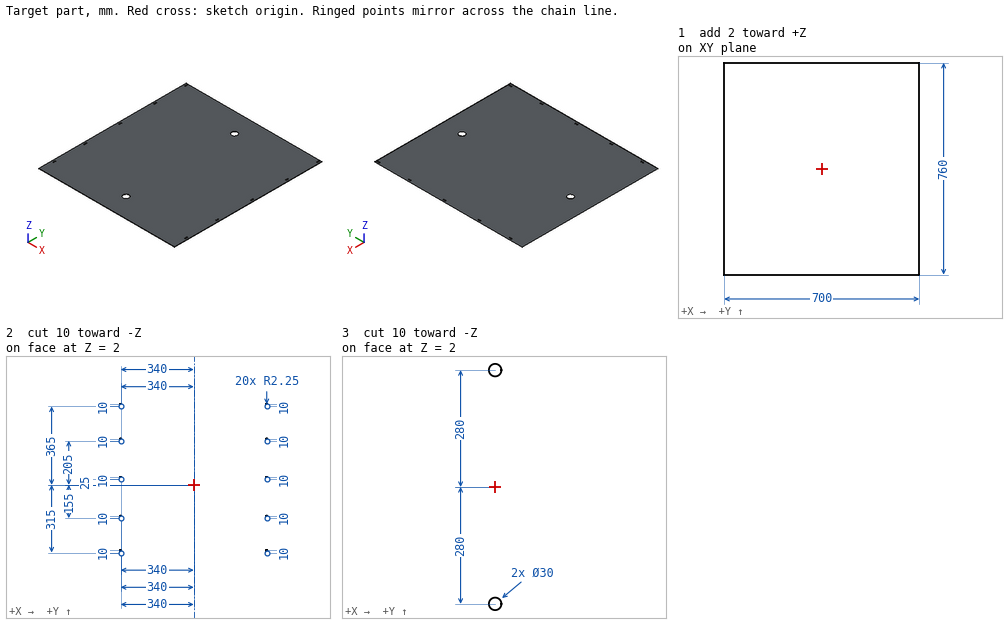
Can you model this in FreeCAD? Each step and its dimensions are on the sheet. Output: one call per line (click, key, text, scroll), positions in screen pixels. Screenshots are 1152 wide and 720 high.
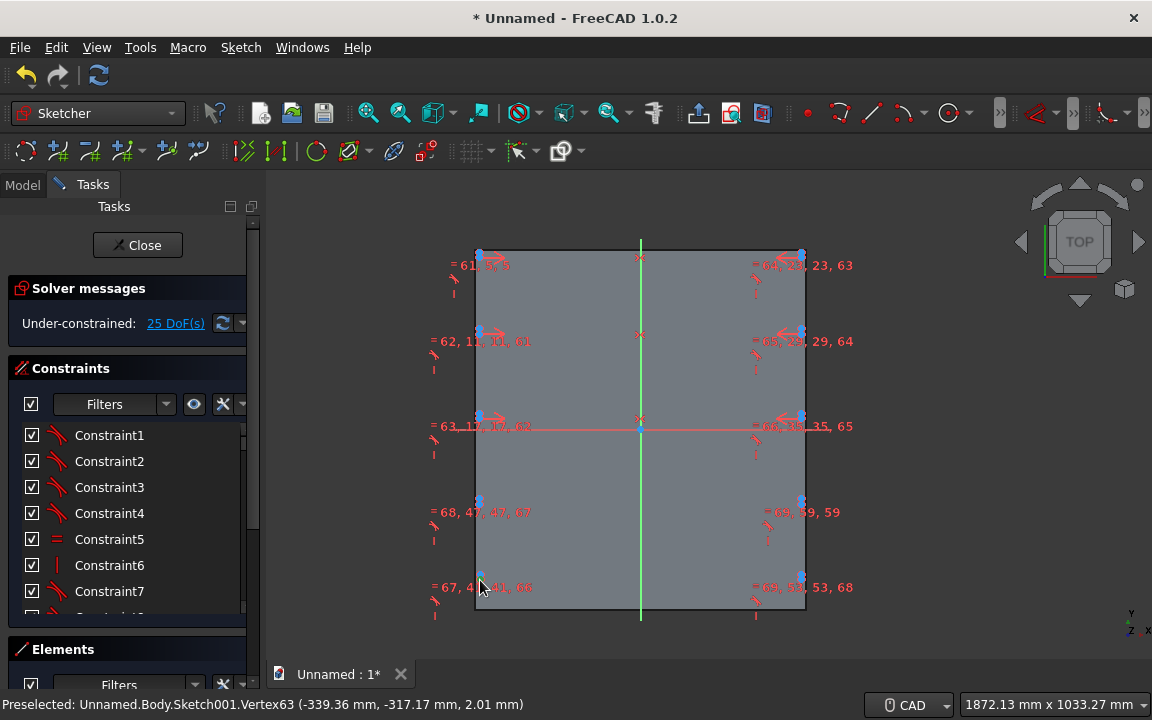
scroll(801, 580, up, 13)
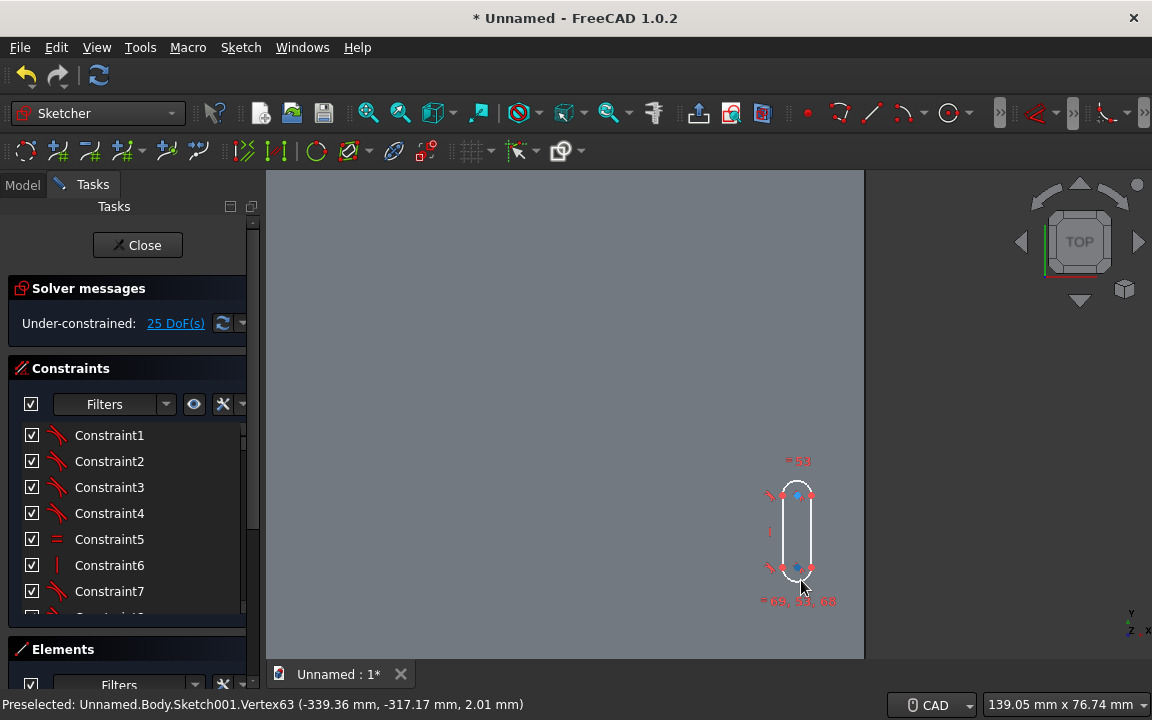
click(797, 567)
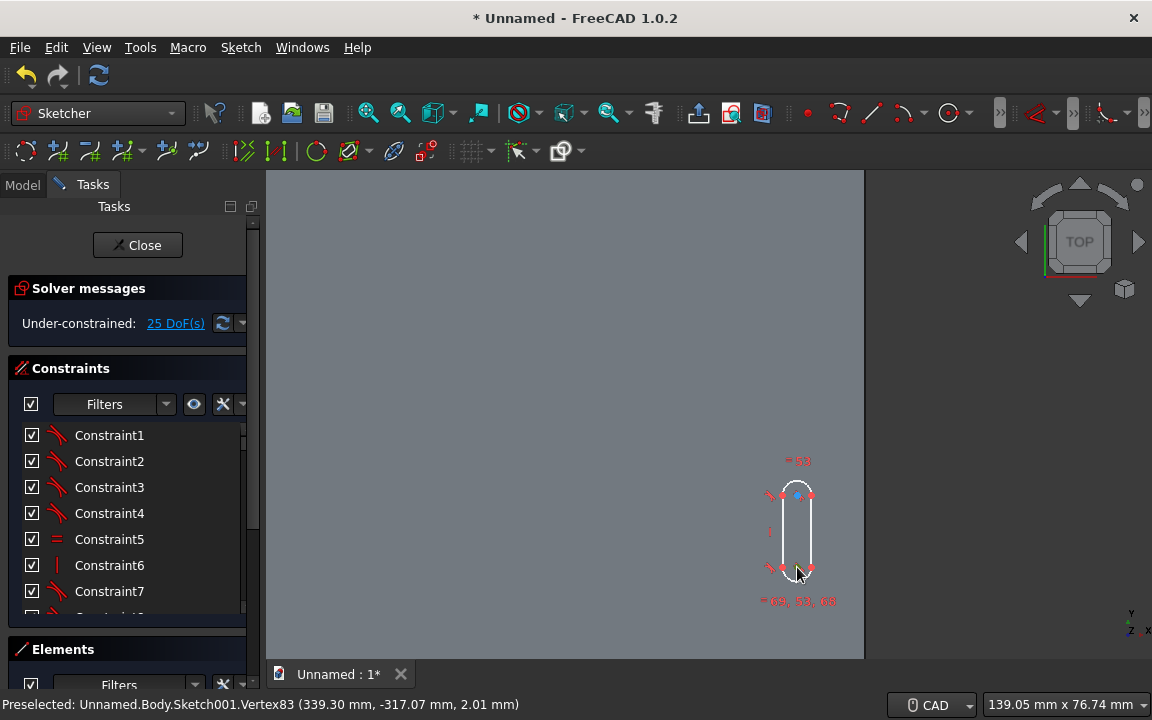
scroll(801, 580, down, 13)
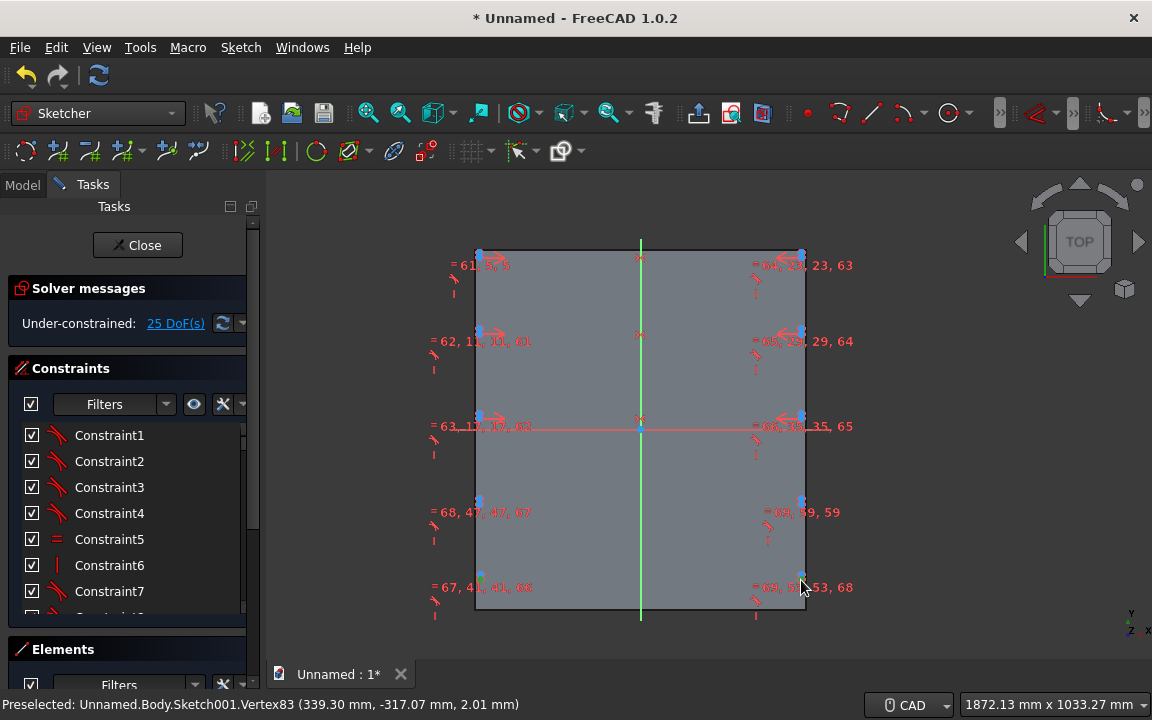
click(641, 600)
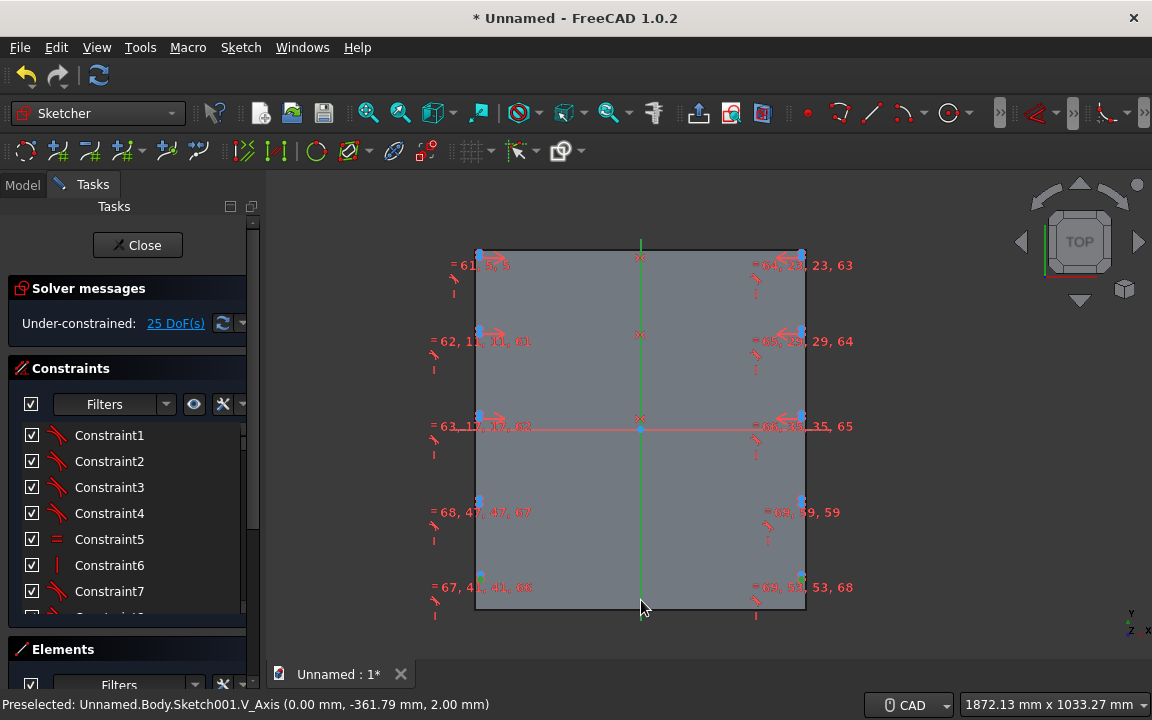
key(s)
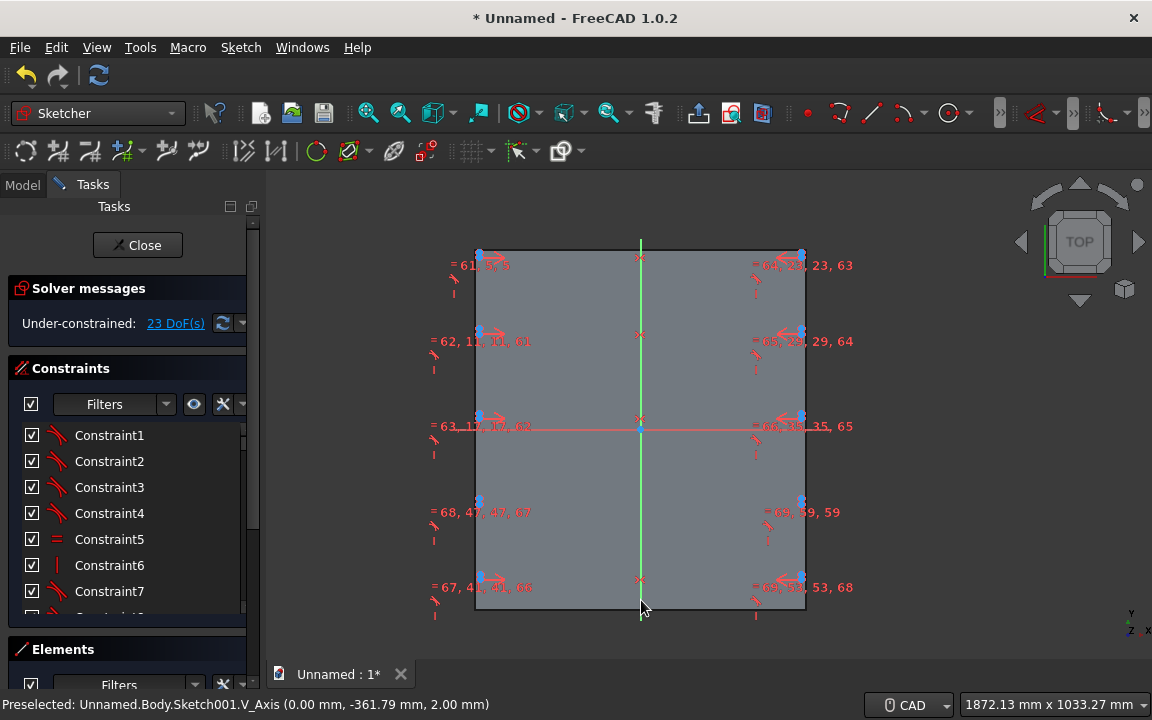
scroll(480, 504, up, 13)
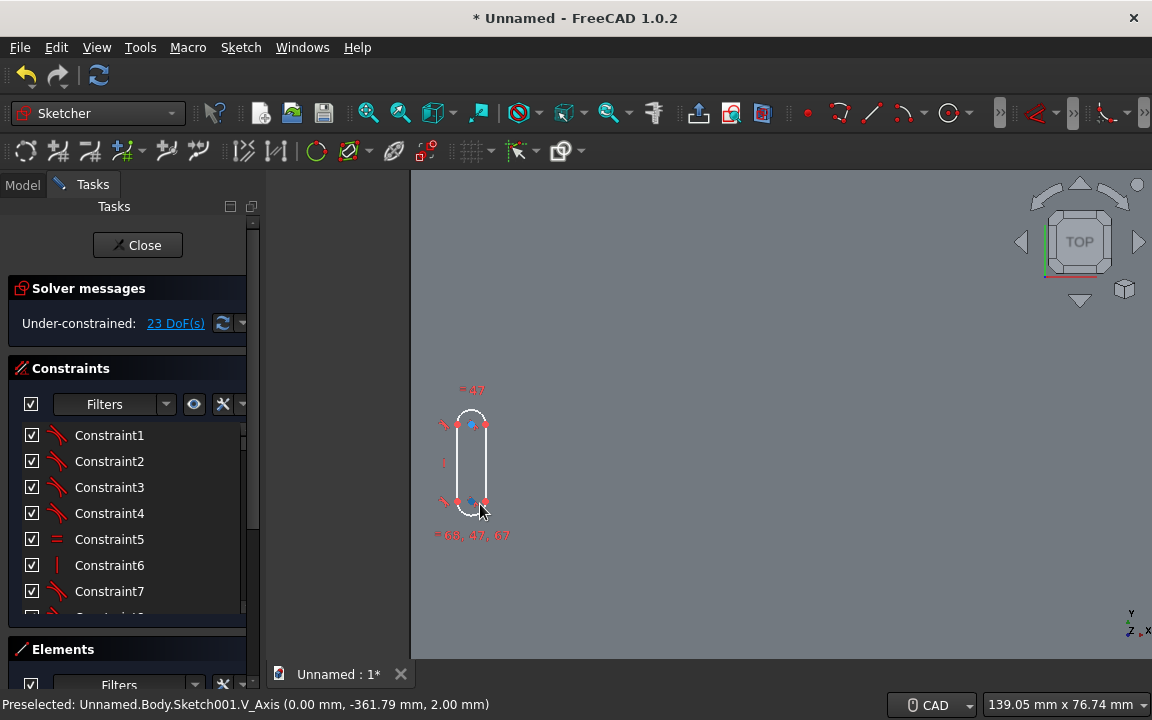
click(471, 501)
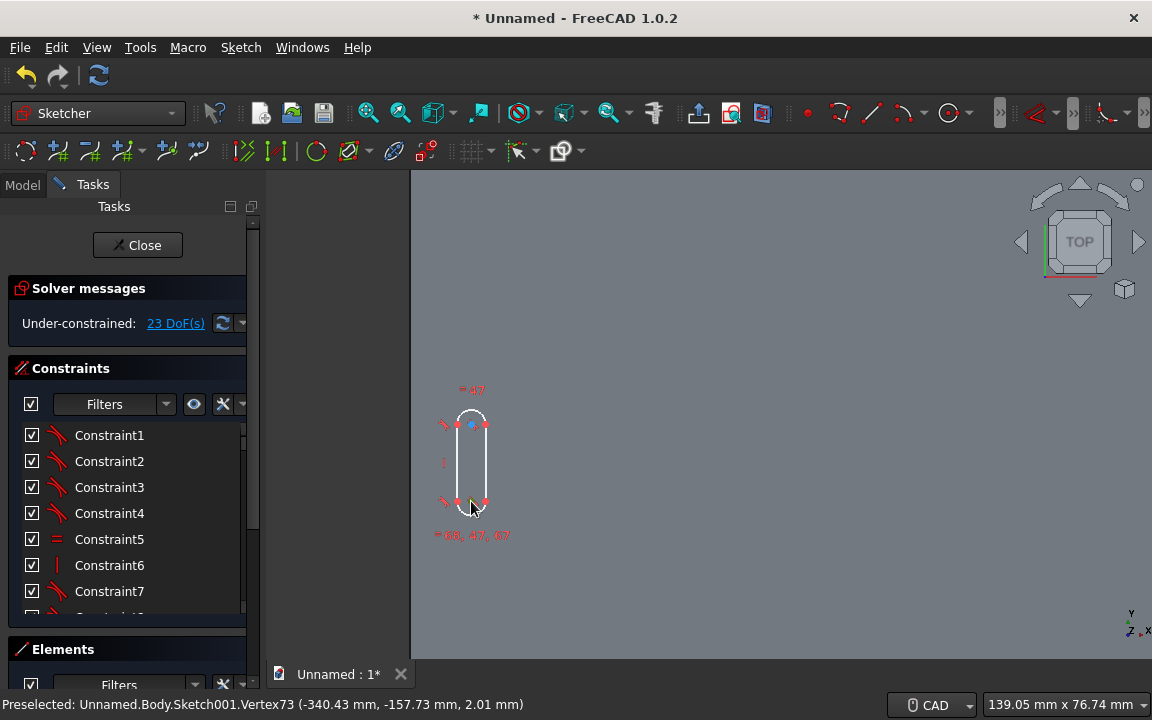
scroll(480, 504, down, 13)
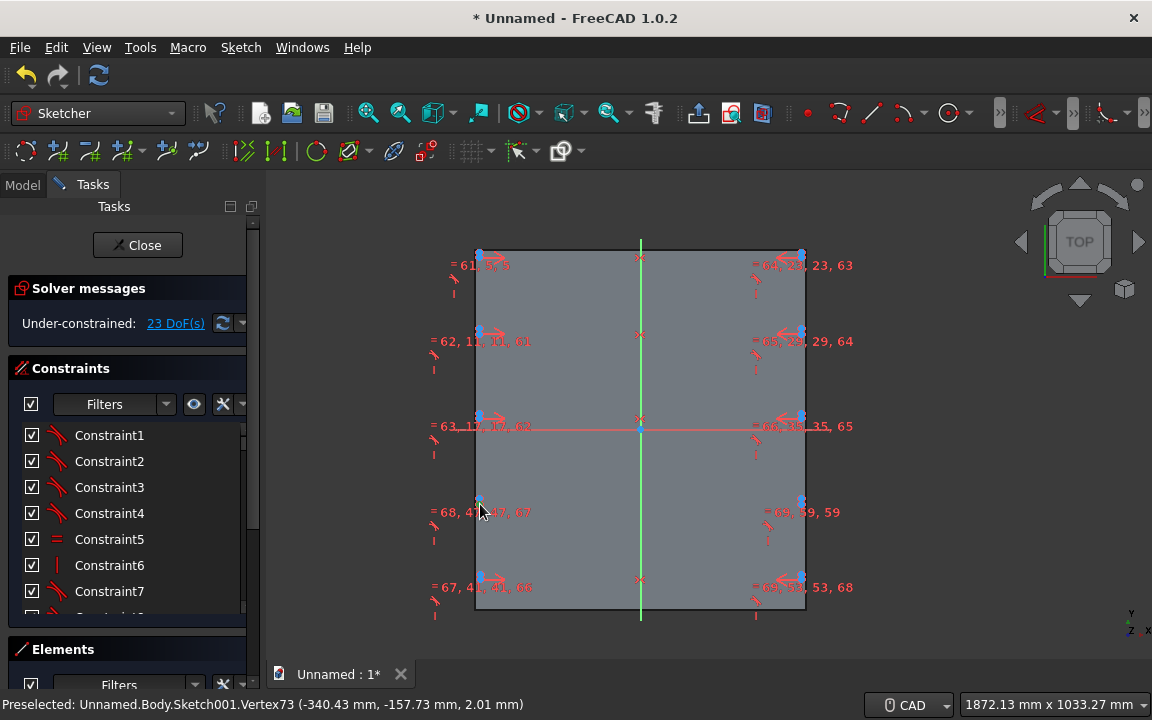
scroll(801, 504, up, 13)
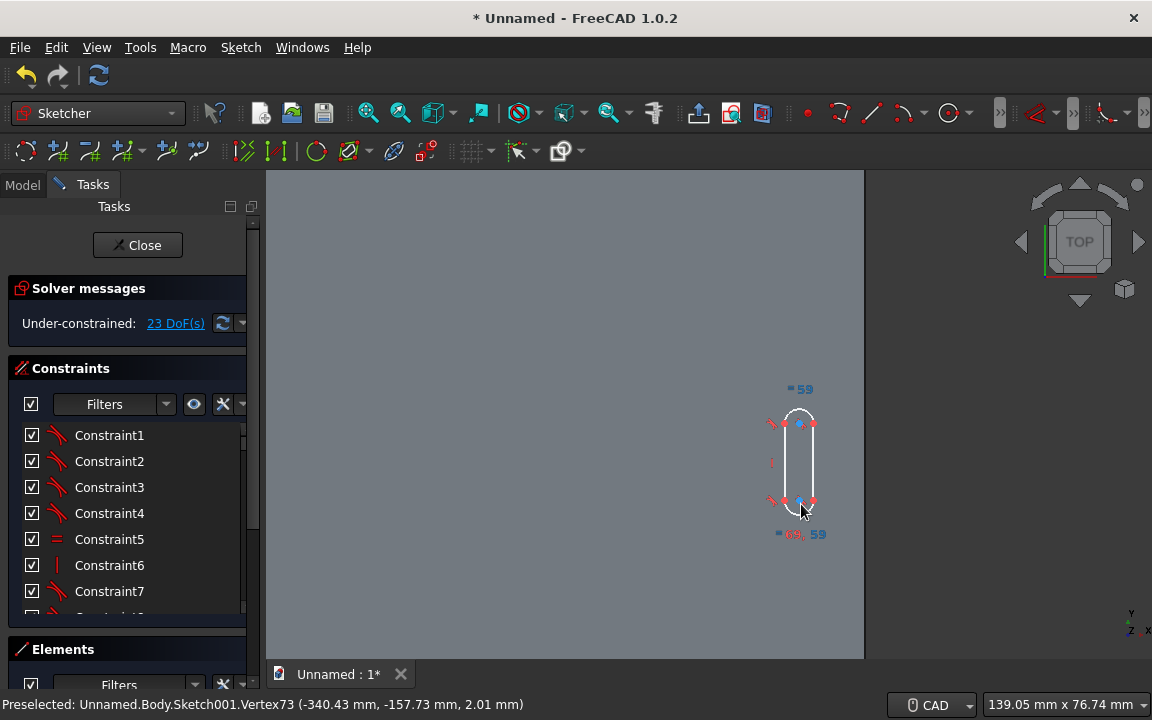
click(799, 501)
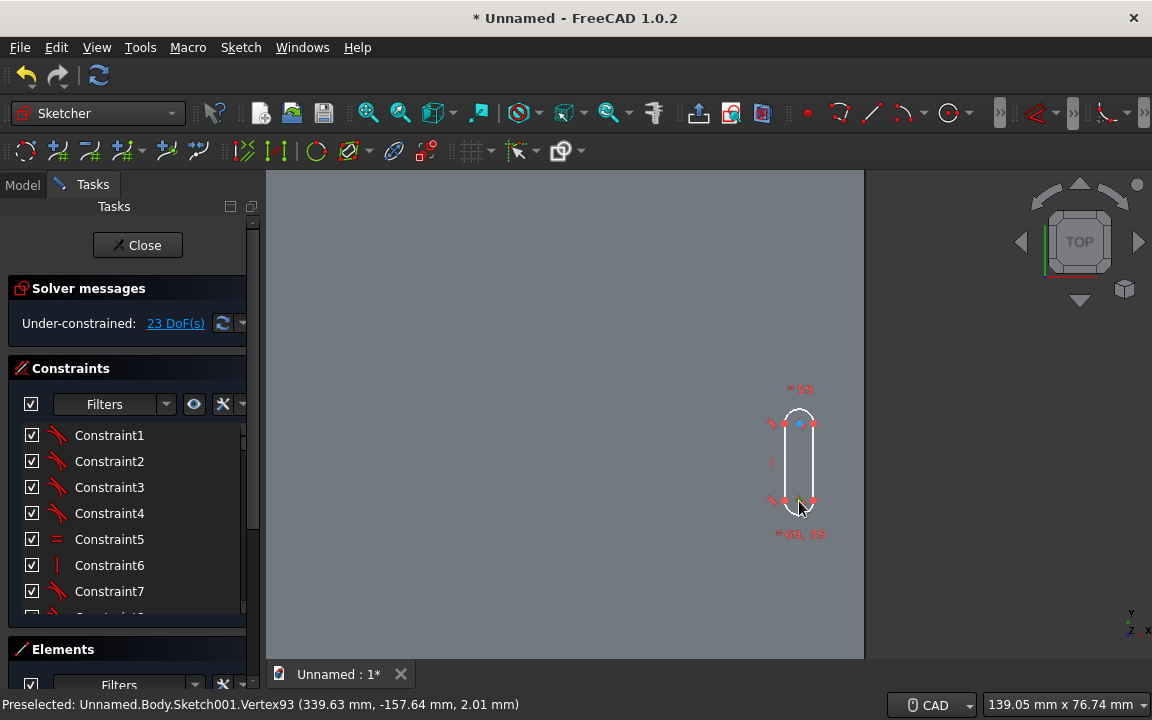
scroll(801, 504, down, 13)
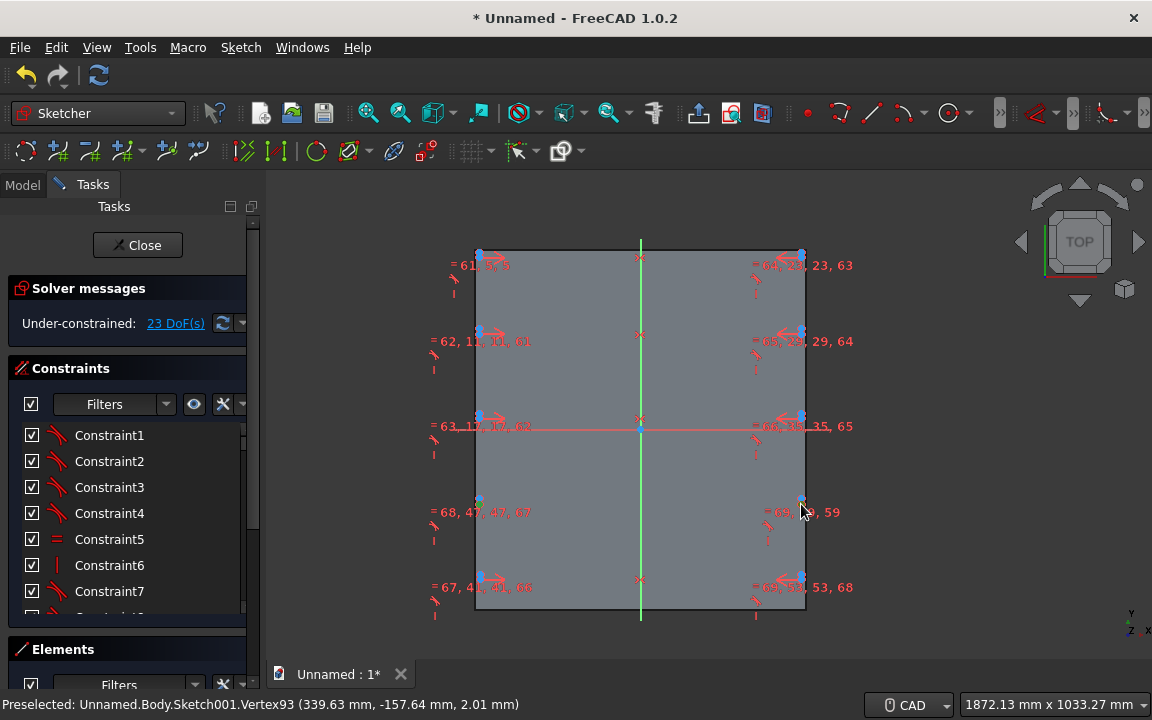
click(641, 600)